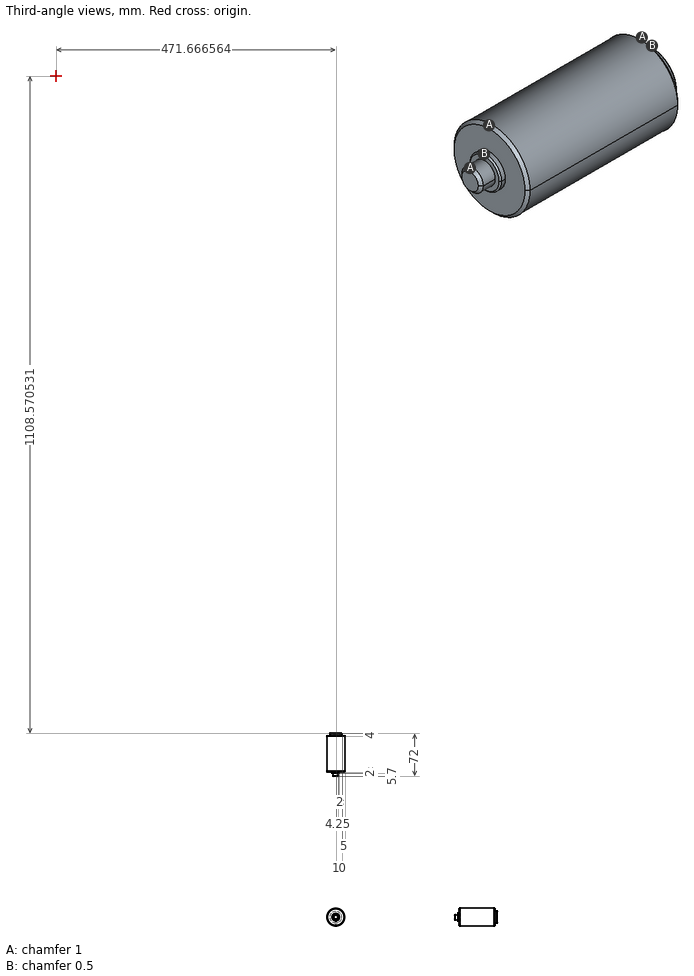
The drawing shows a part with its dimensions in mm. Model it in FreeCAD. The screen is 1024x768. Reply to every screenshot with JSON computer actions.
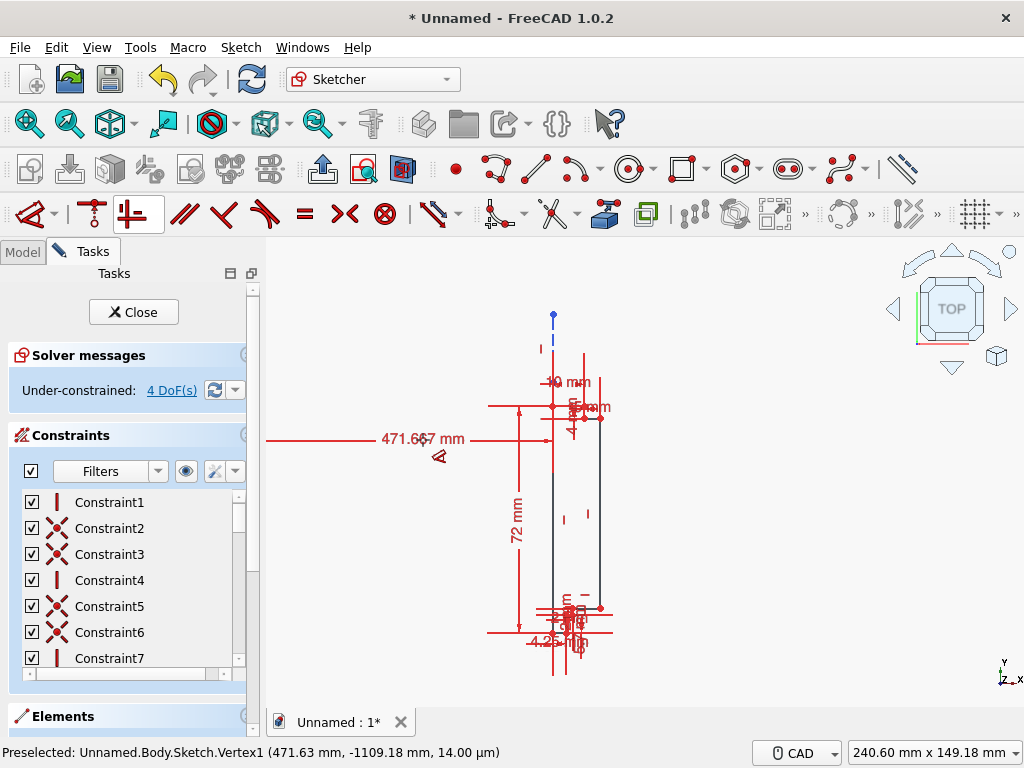
{"action": "left_click", "coordinate": [553, 382]}
{"action": "left_click", "coordinate": [424, 416]}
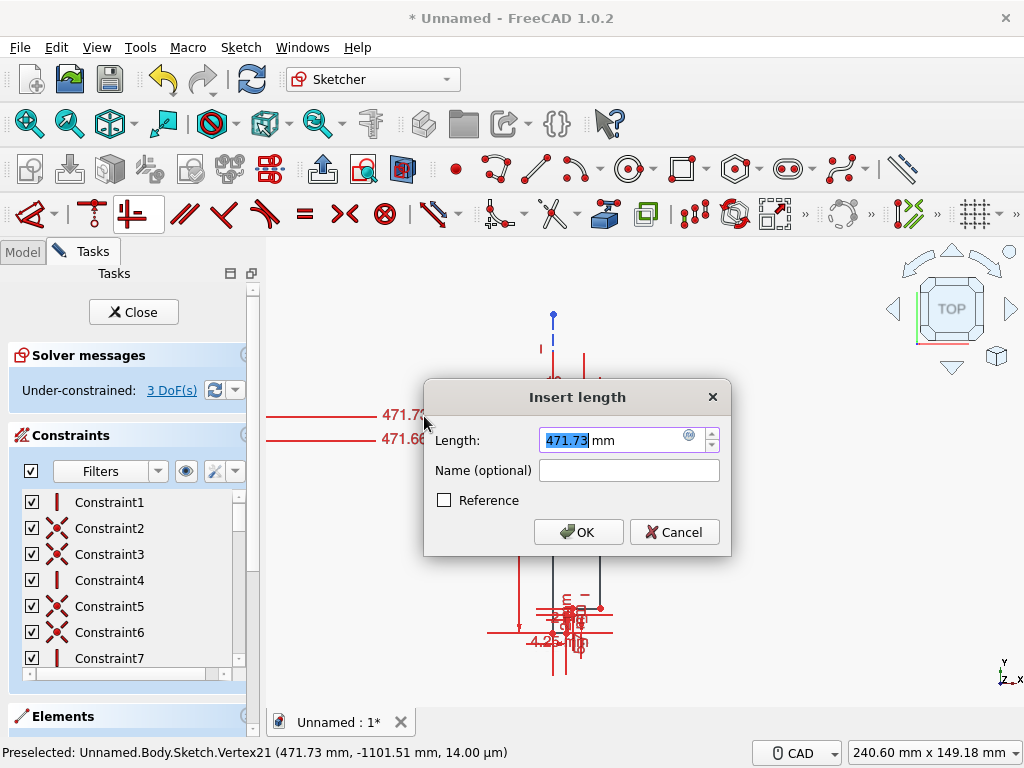
{"action": "type", "text": "471.666564"}
{"action": "key", "text": "Return"}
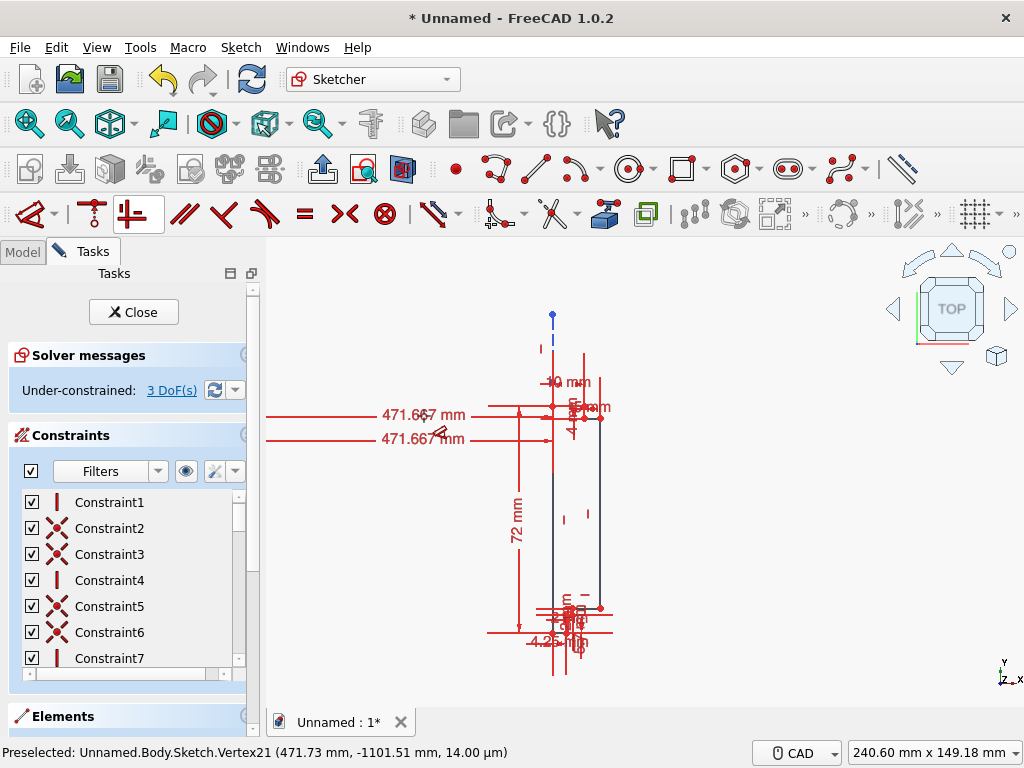
{"action": "left_click", "coordinate": [553, 406]}
{"action": "left_click", "coordinate": [587, 336]}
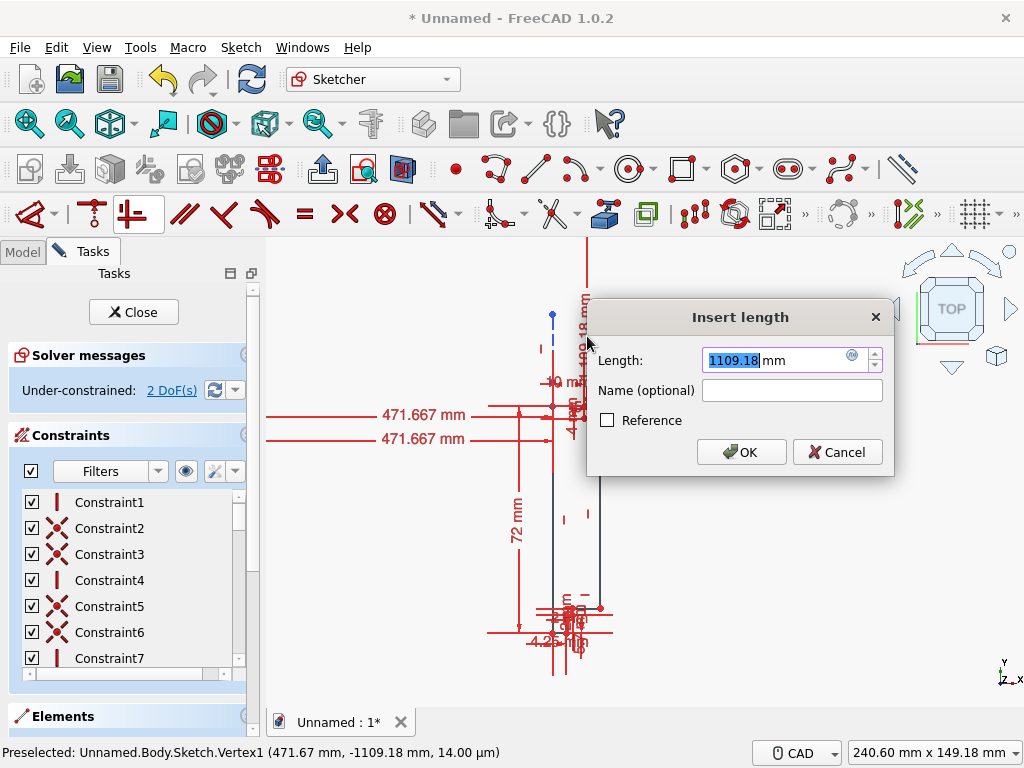
{"action": "type", "text": "1108.570531"}
{"action": "key", "text": "Return"}
{"action": "key", "text": "Escape"}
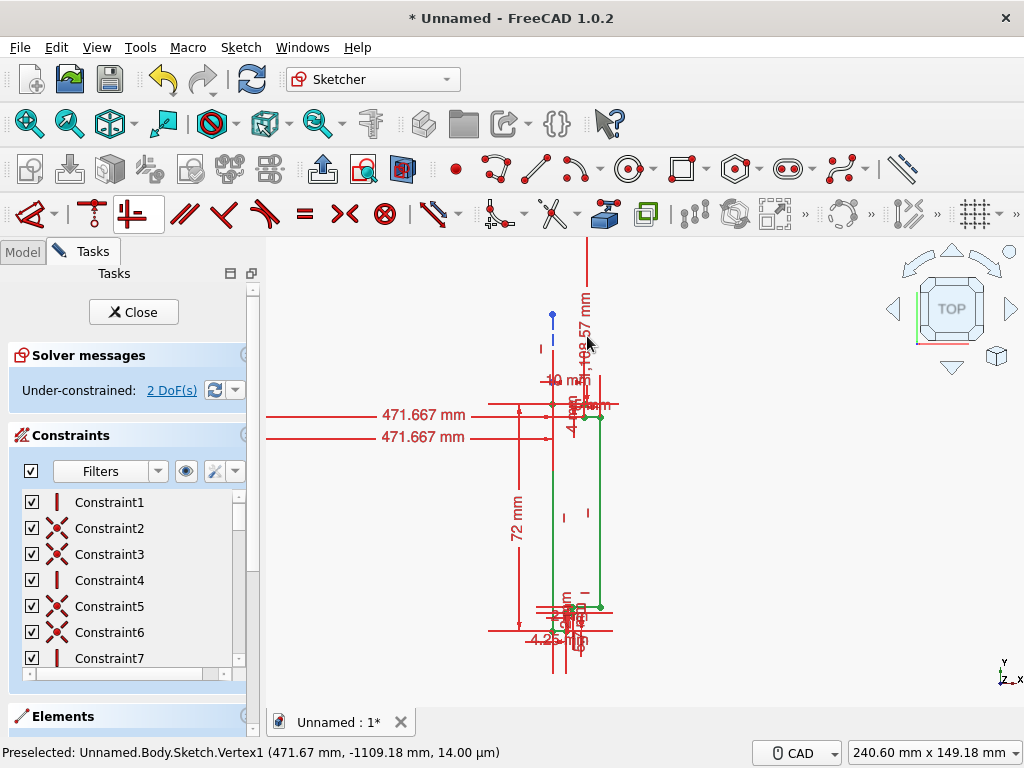
{"action": "left_click", "coordinate": [134, 312]}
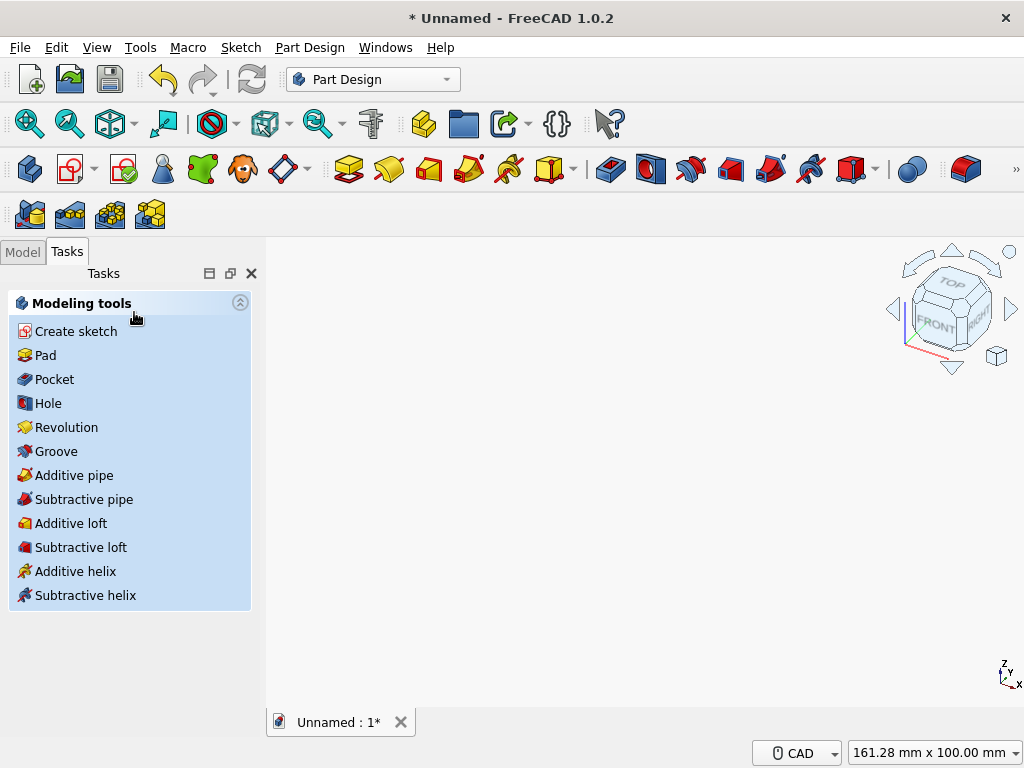
{"action": "left_click", "coordinate": [390, 170]}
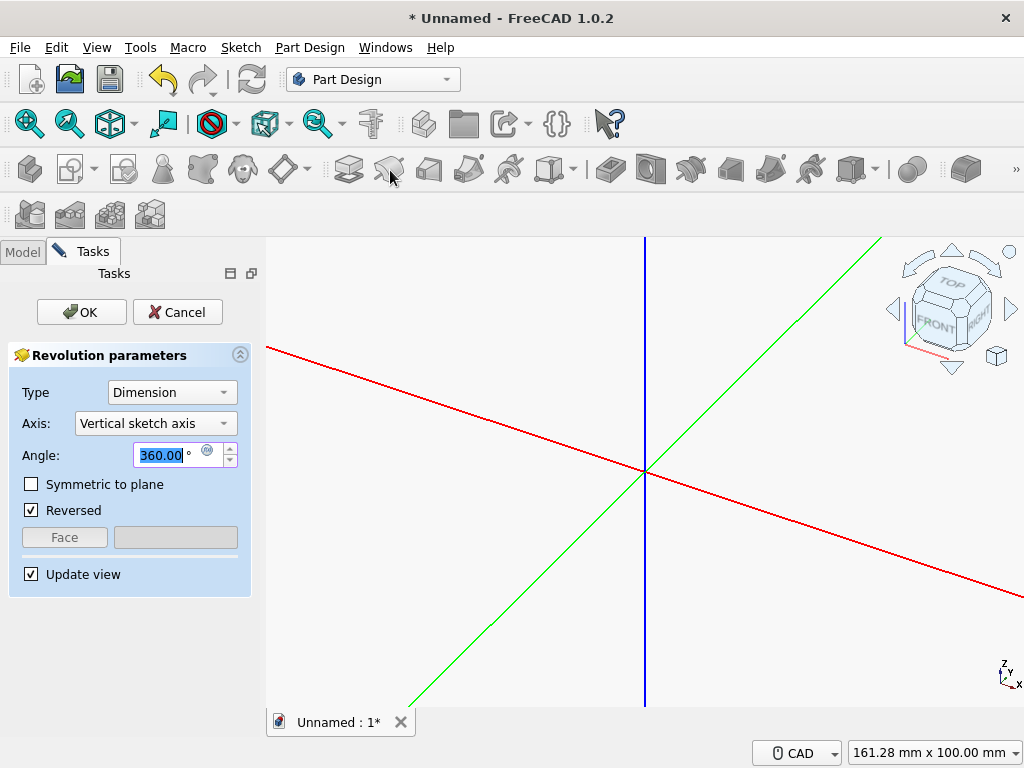
{"action": "left_click", "coordinate": [156, 424]}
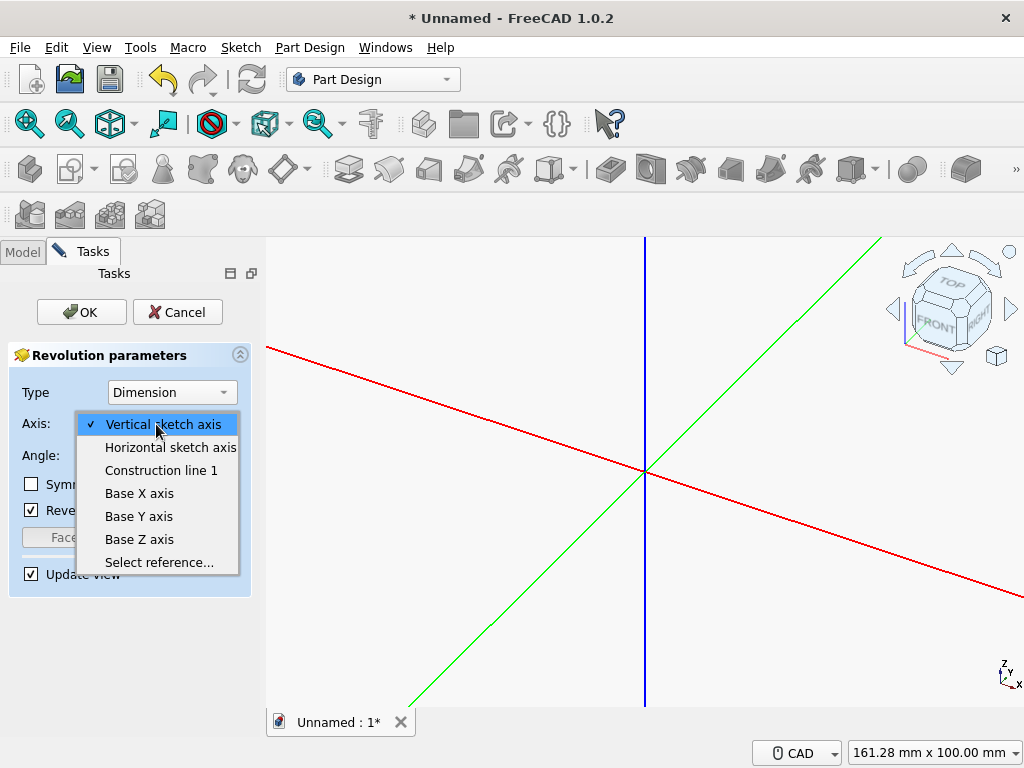
{"action": "left_click", "coordinate": [156, 470]}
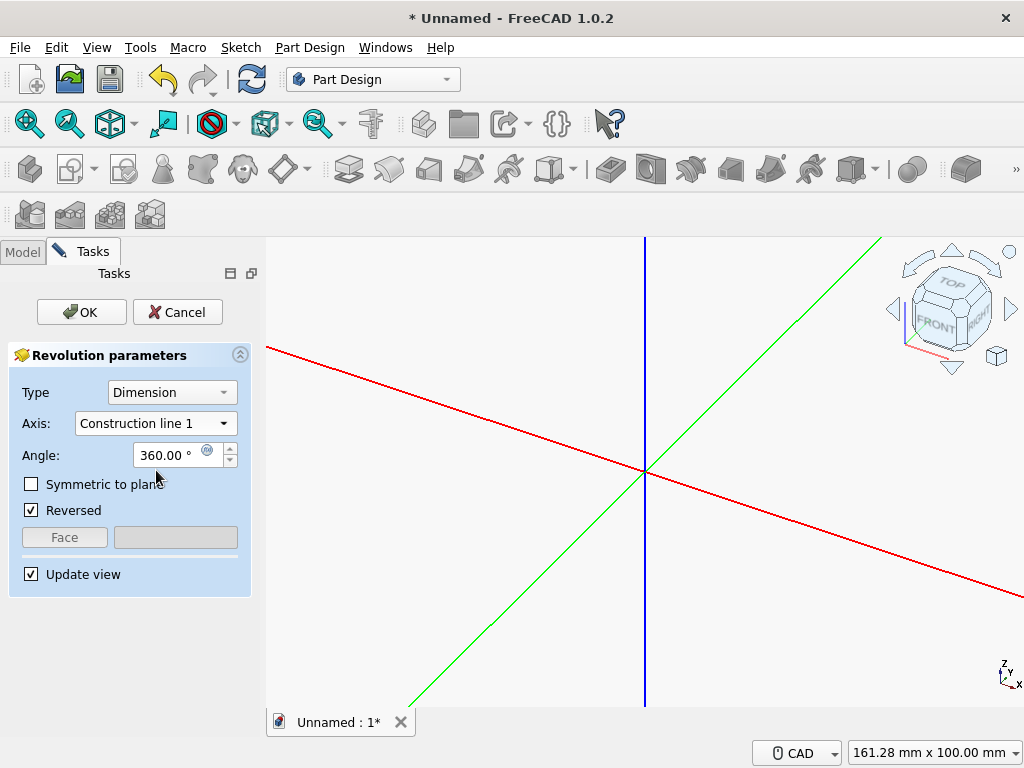
{"action": "left_click", "coordinate": [82, 312]}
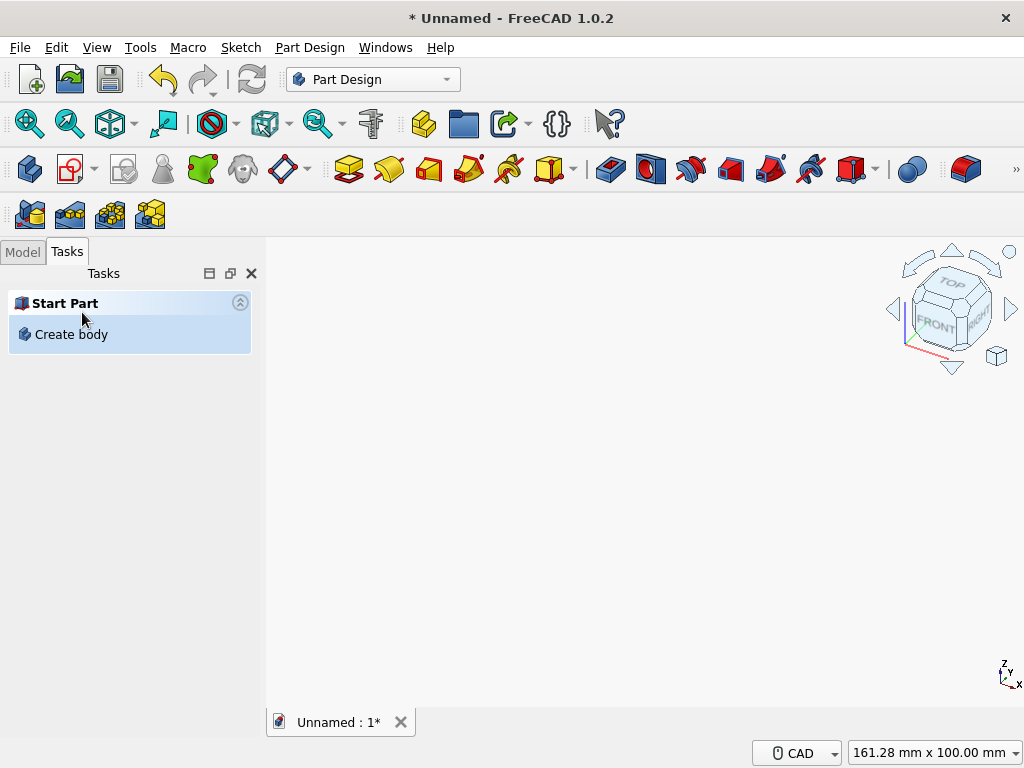
{"action": "key", "text": "v f"}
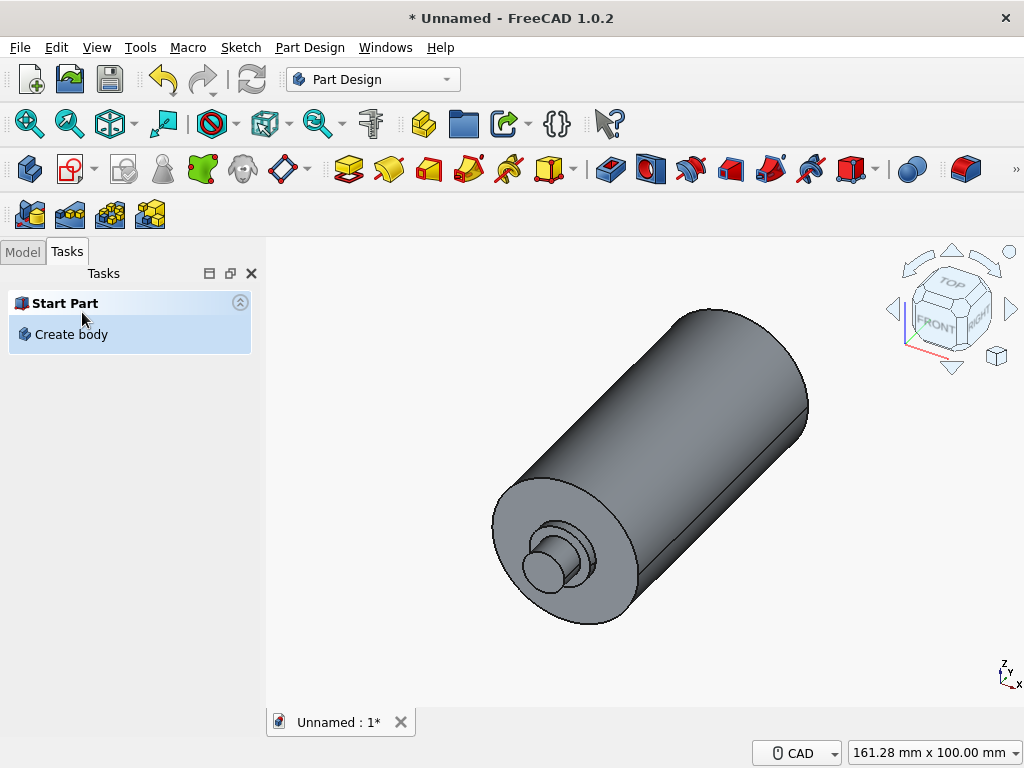
{"action": "left_click", "coordinate": [506, 490]}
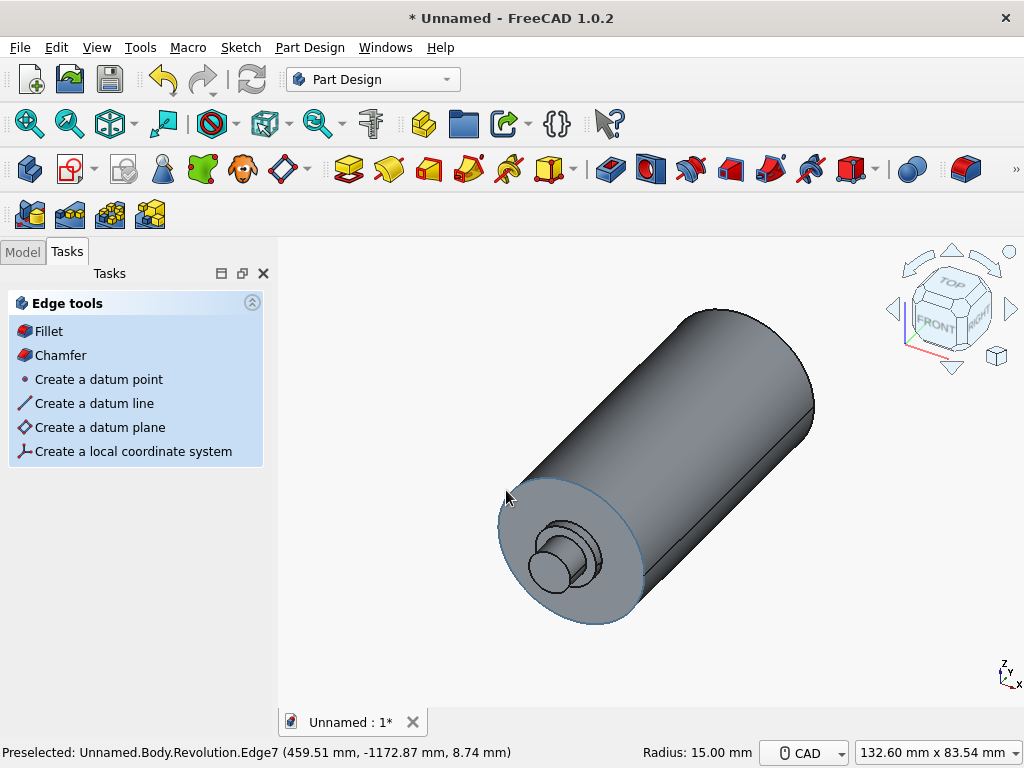
{"action": "left_click", "coordinate": [529, 565], "text": "ctrl"}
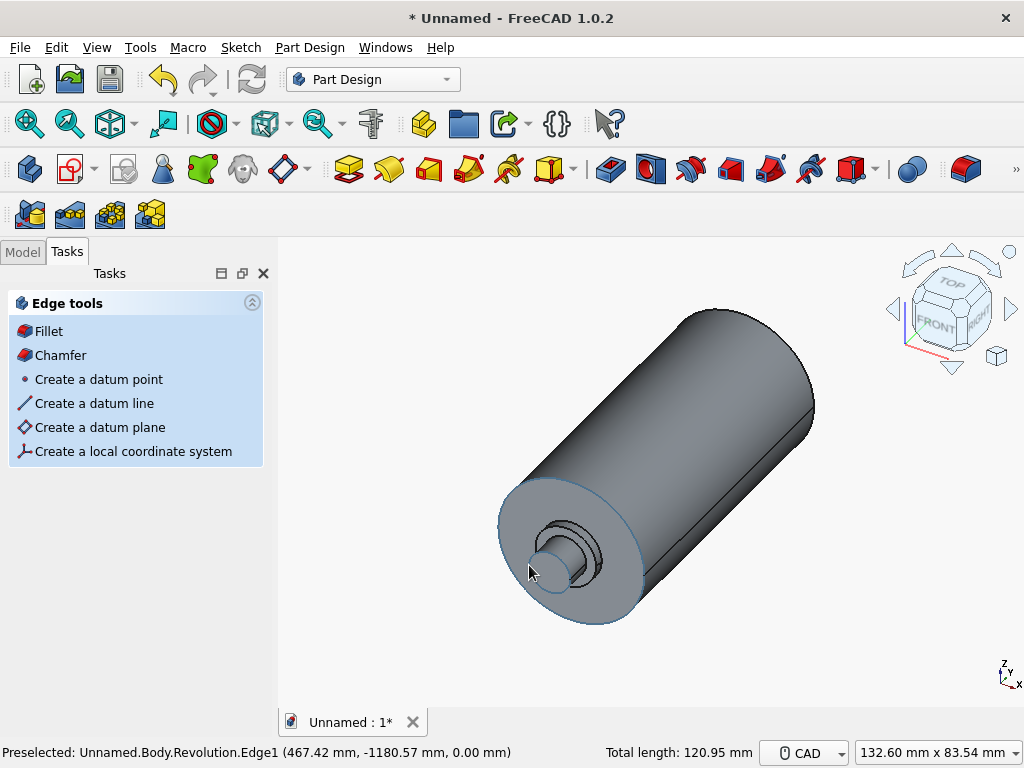
{"action": "key", "text": "0"}